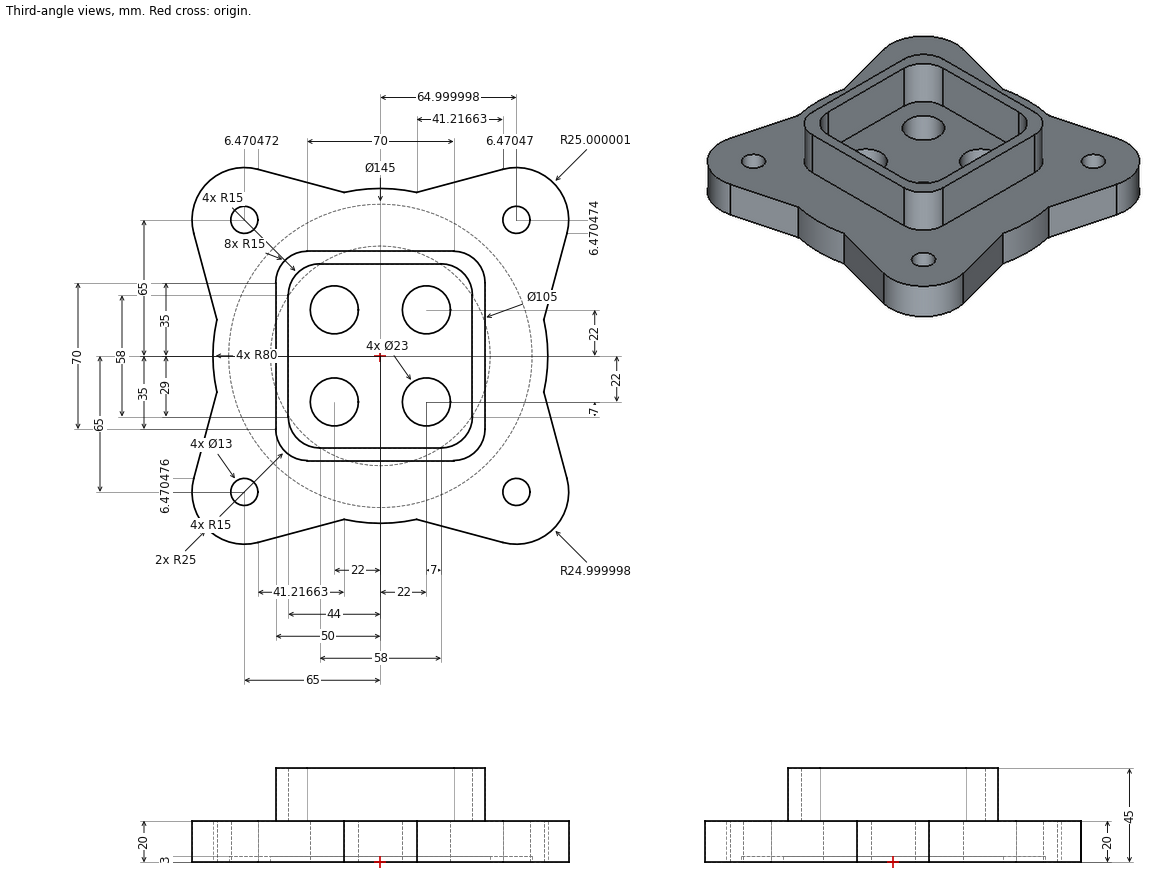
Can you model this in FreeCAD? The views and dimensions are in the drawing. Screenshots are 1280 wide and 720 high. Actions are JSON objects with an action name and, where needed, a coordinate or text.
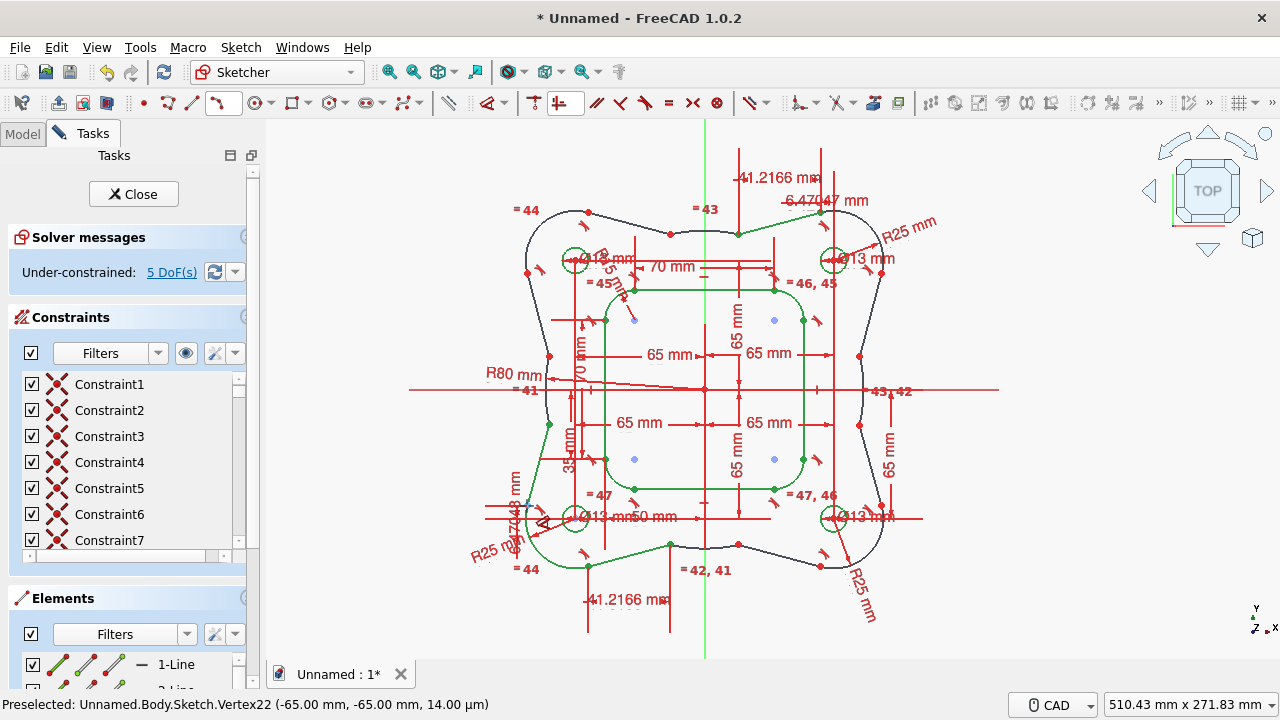
{"action": "scroll", "coordinate": [821, 567], "scroll_direction": "up", "scroll_amount": 6}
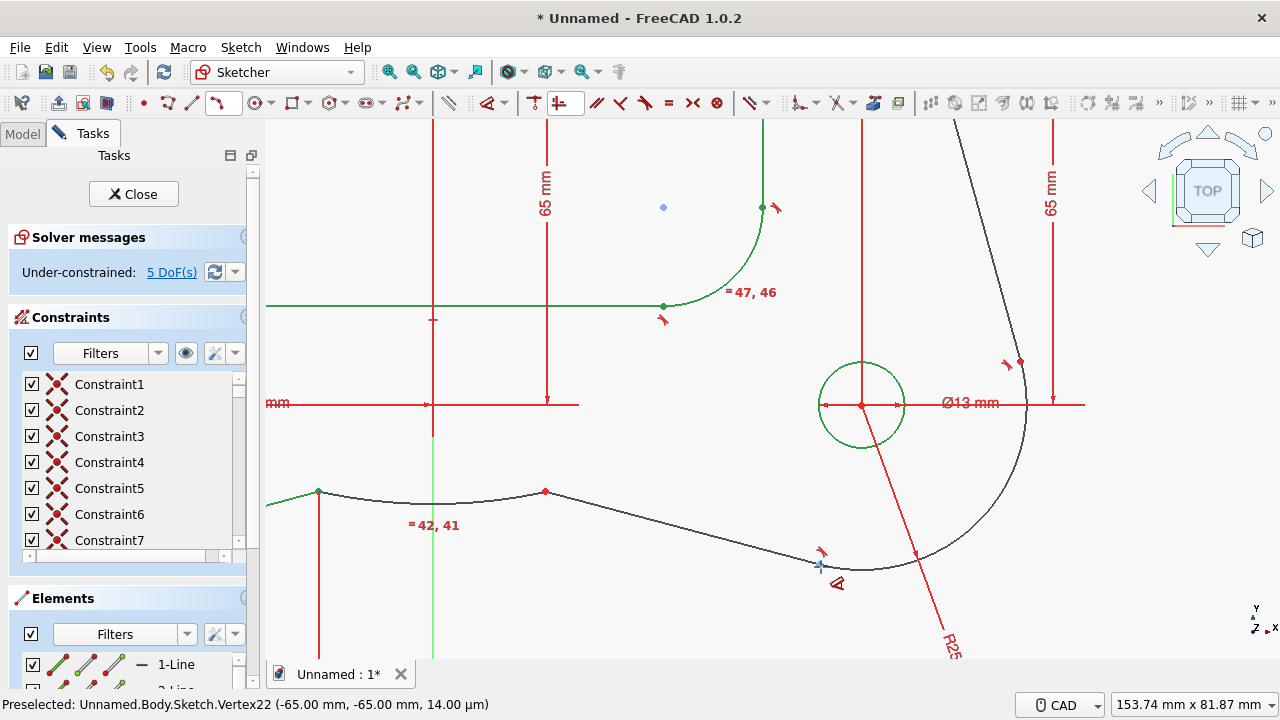
{"action": "left_click", "coordinate": [819, 564]}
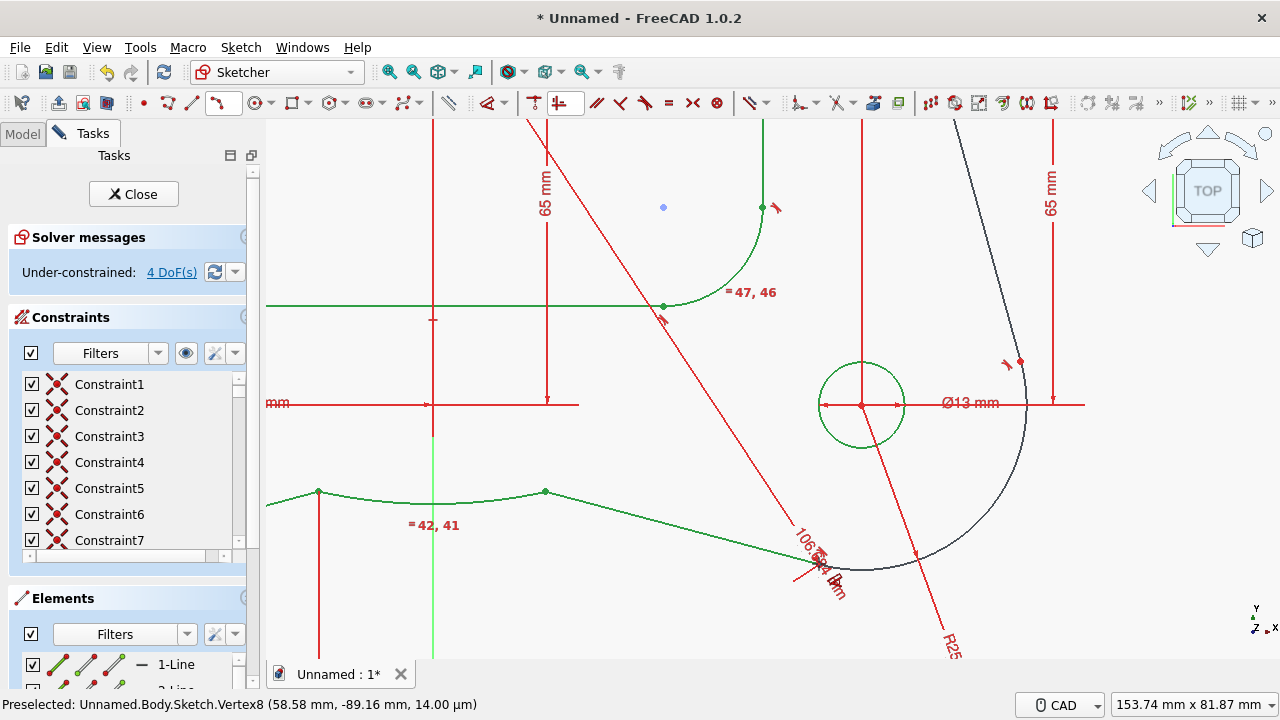
{"action": "left_click", "coordinate": [862, 405]}
{"action": "left_click", "coordinate": [841, 598]}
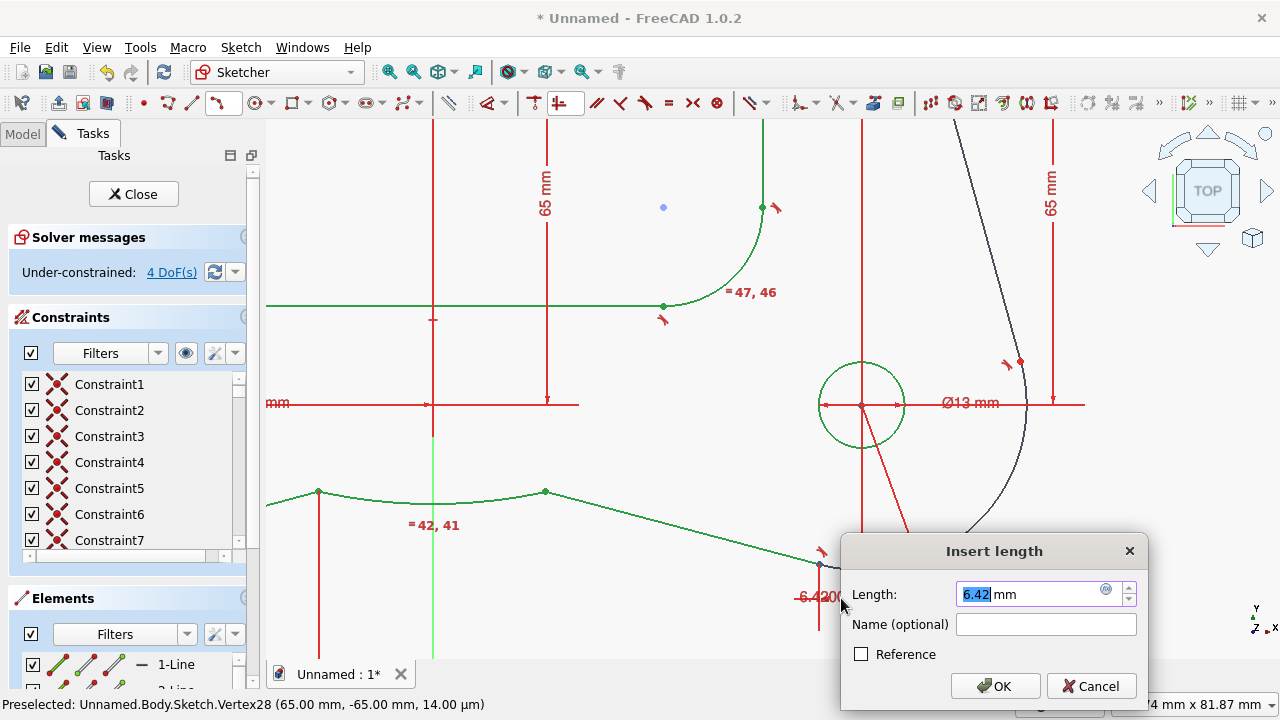
{"action": "type", "text": "6.470475"}
{"action": "key", "text": "Return"}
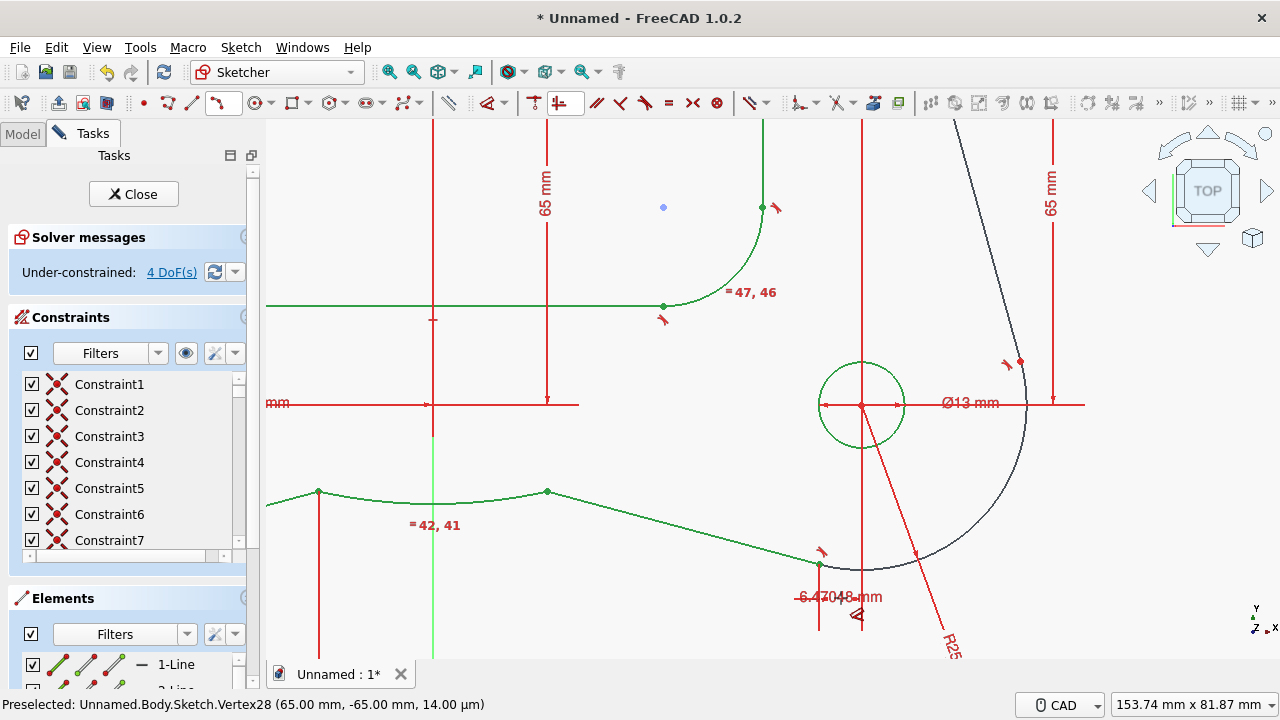
{"action": "left_click", "coordinate": [1021, 361]}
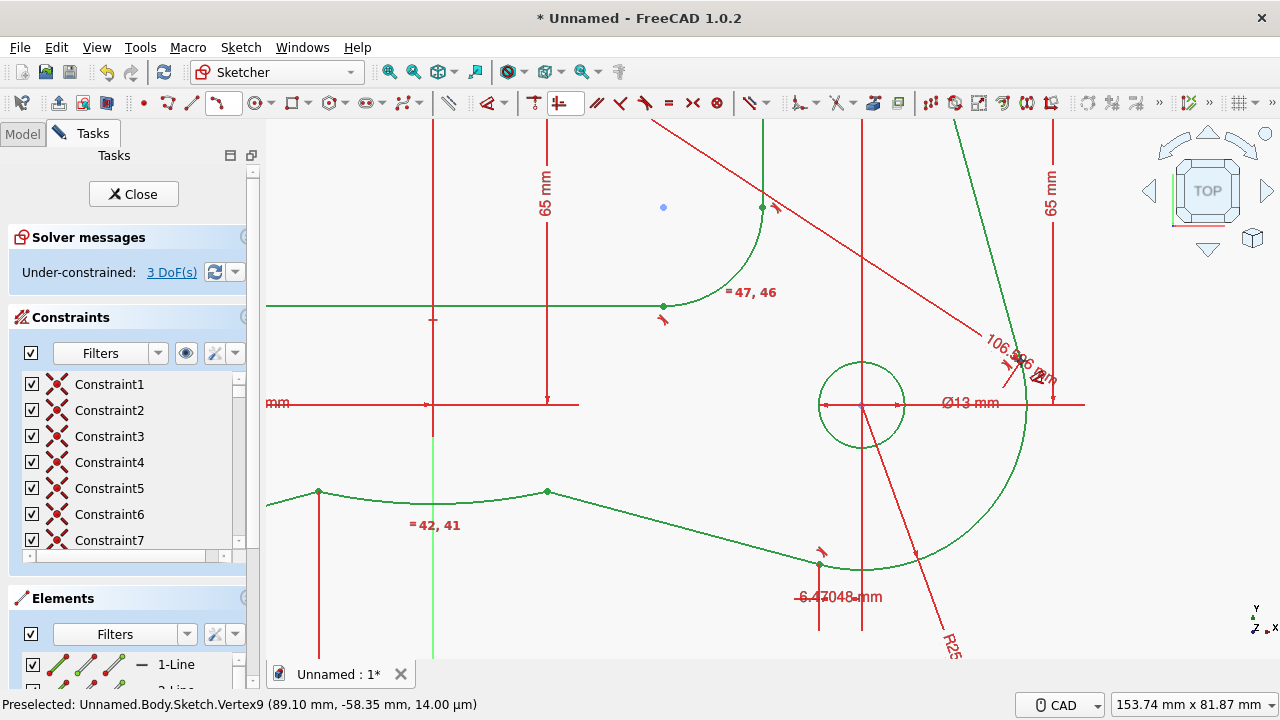
{"action": "left_click", "coordinate": [862, 405]}
{"action": "left_click", "coordinate": [1055, 383]}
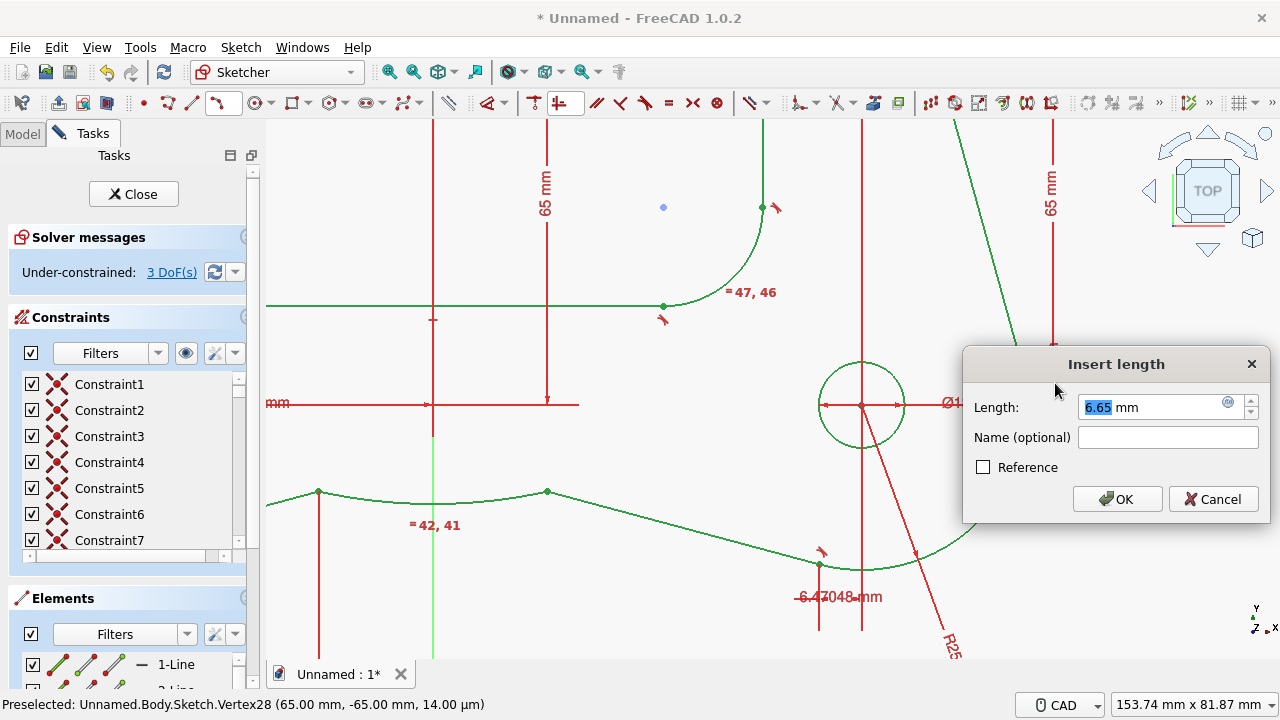
{"action": "type", "text": "6.470479"}
{"action": "key", "text": "Return"}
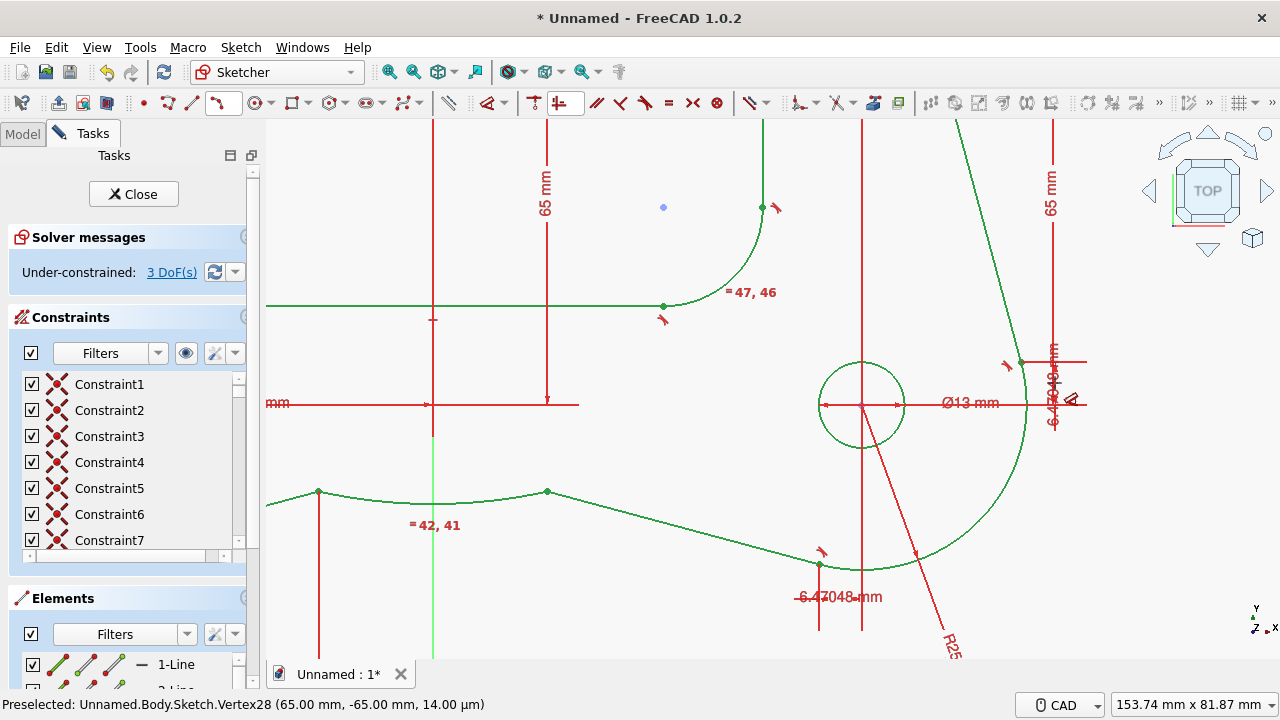
{"action": "scroll", "coordinate": [822, 567], "scroll_direction": "down", "scroll_amount": 6}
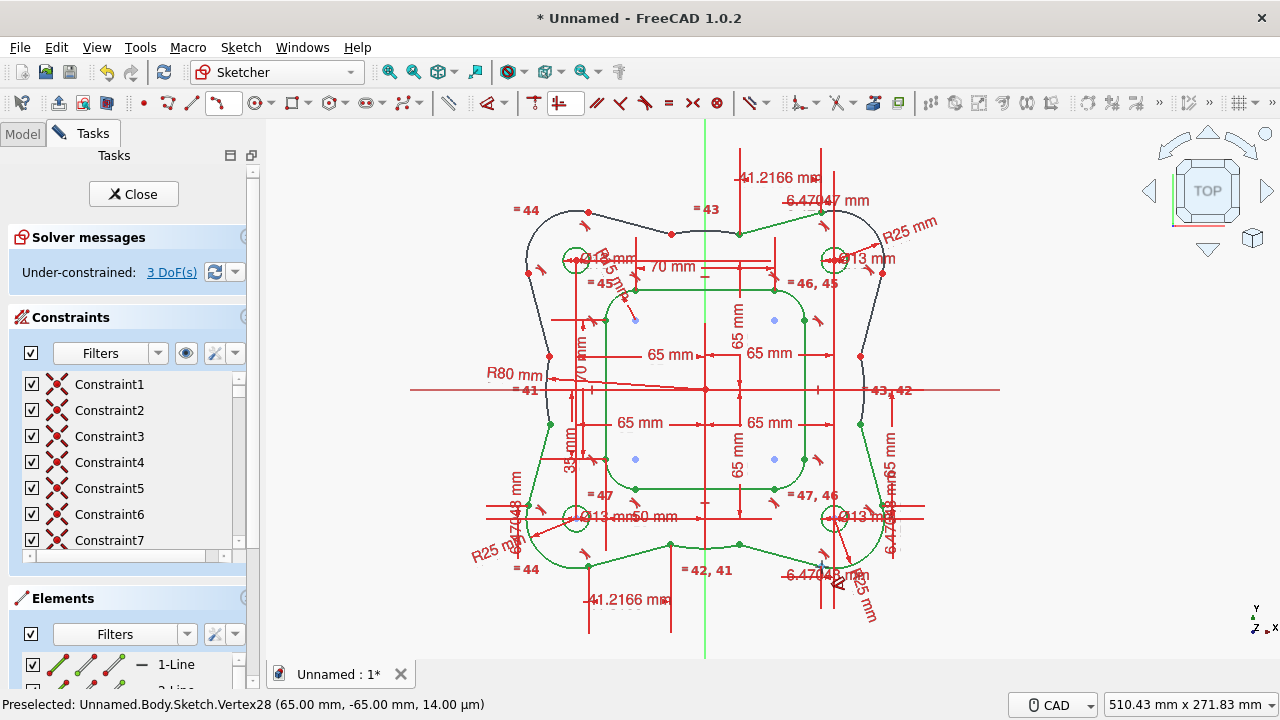
{"action": "scroll", "coordinate": [589, 213], "scroll_direction": "up", "scroll_amount": 6}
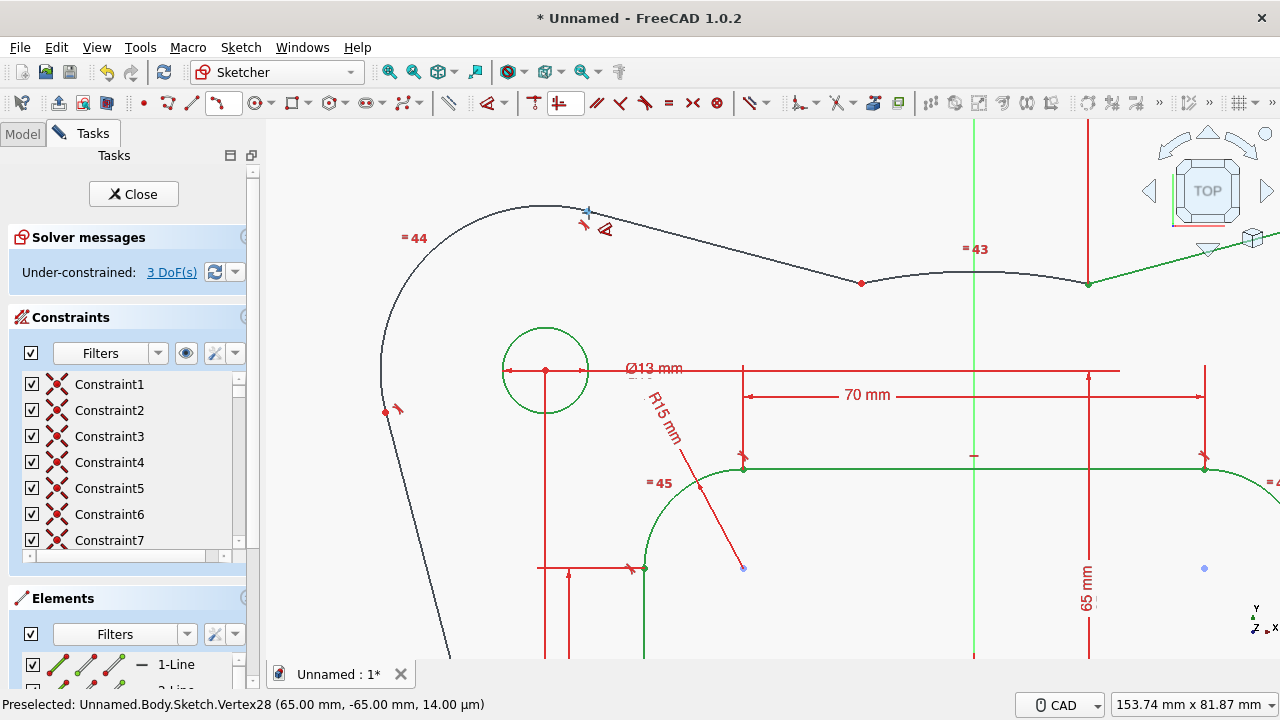
{"action": "left_click", "coordinate": [588, 211]}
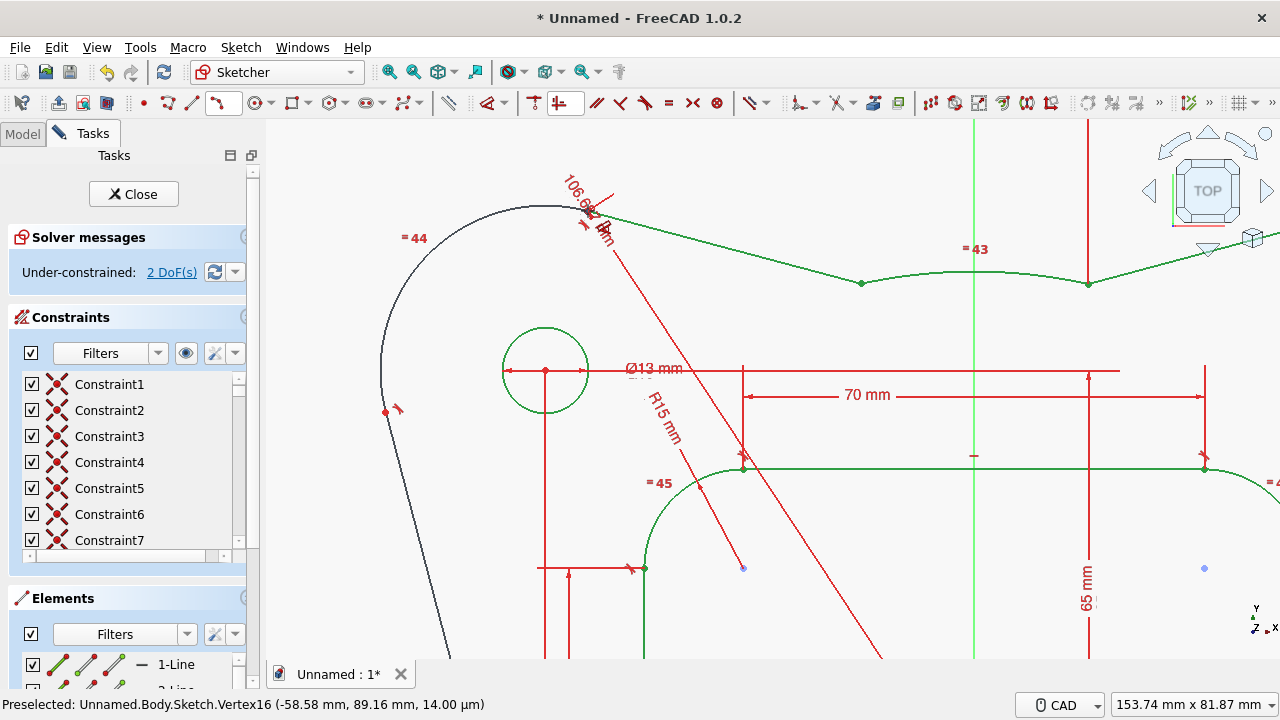
{"action": "left_click", "coordinate": [545, 371]}
{"action": "left_click", "coordinate": [567, 177]}